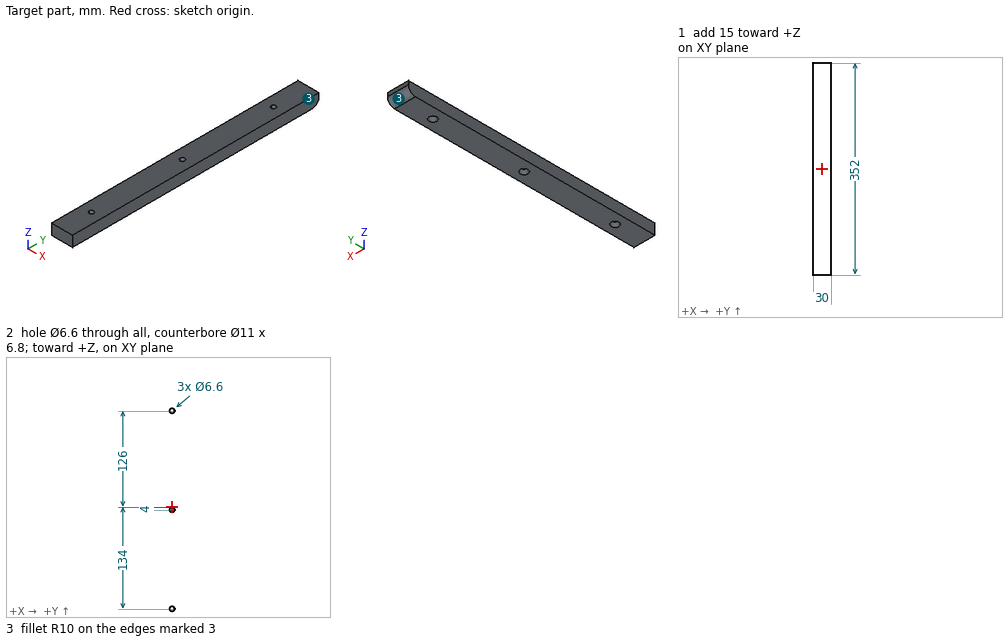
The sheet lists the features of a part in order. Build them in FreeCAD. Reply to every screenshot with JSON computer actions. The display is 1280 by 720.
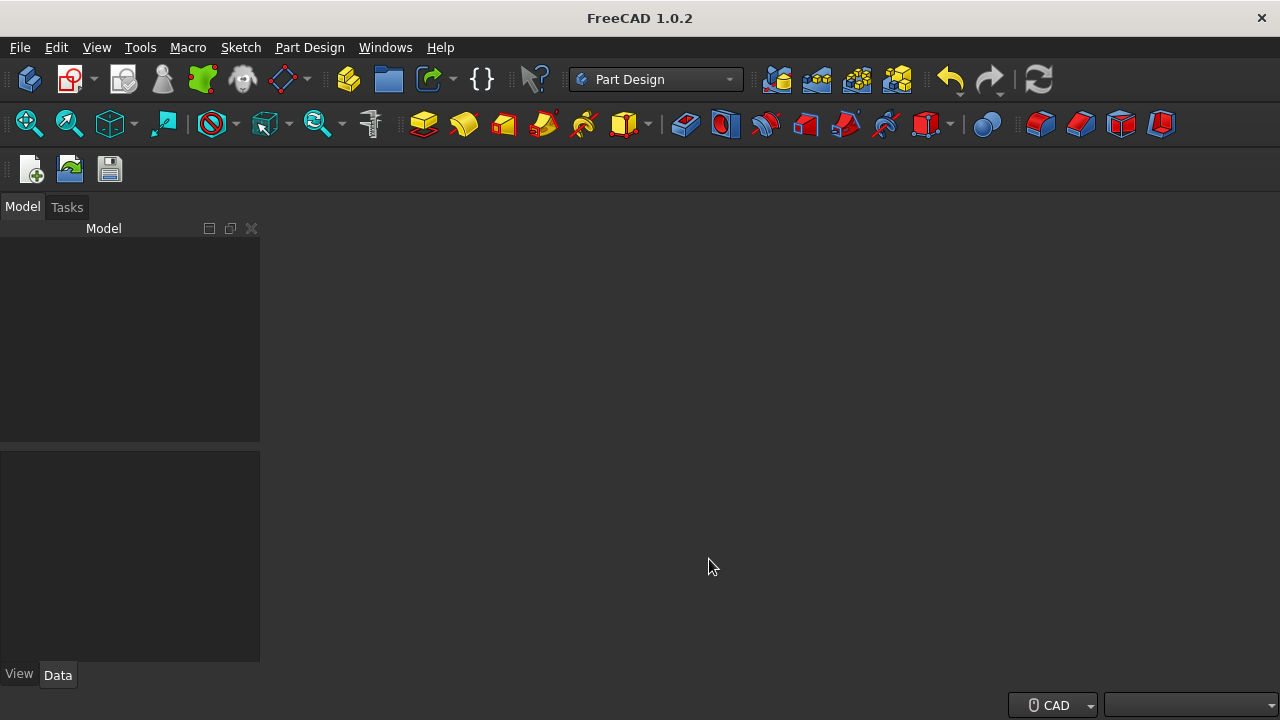
{"action": "left_click", "coordinate": [30, 170]}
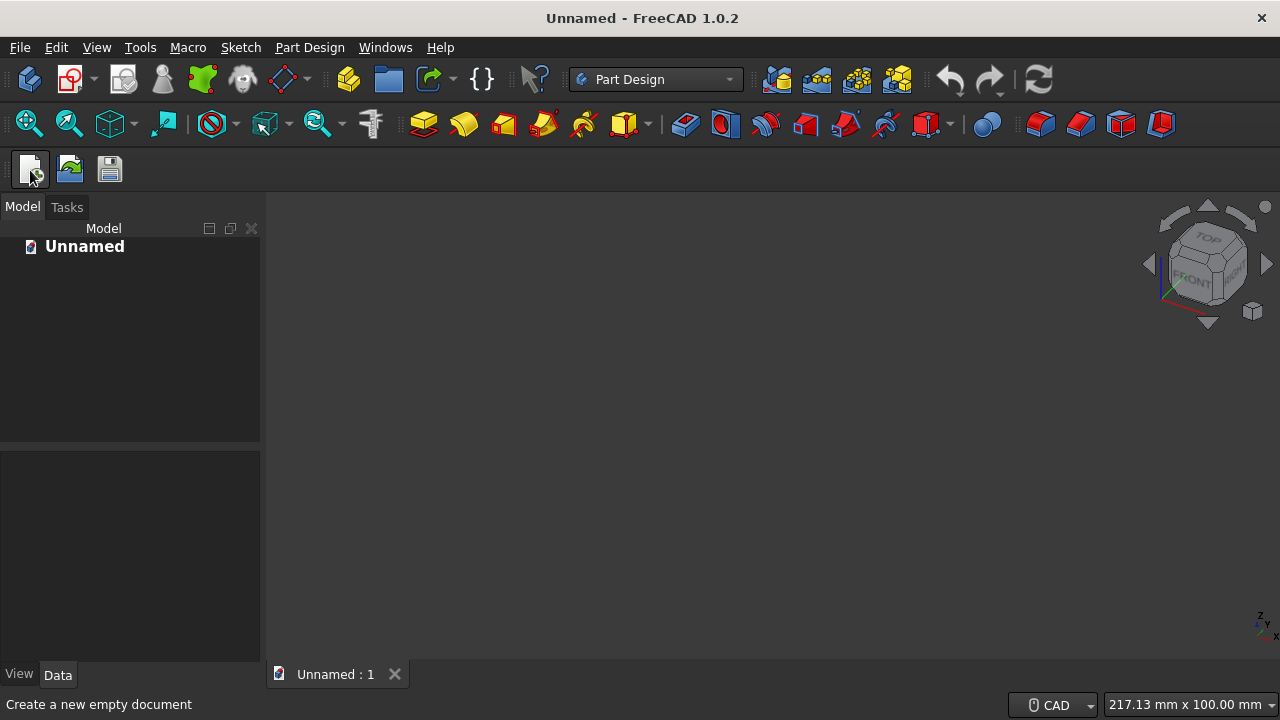
{"action": "left_click", "coordinate": [70, 80]}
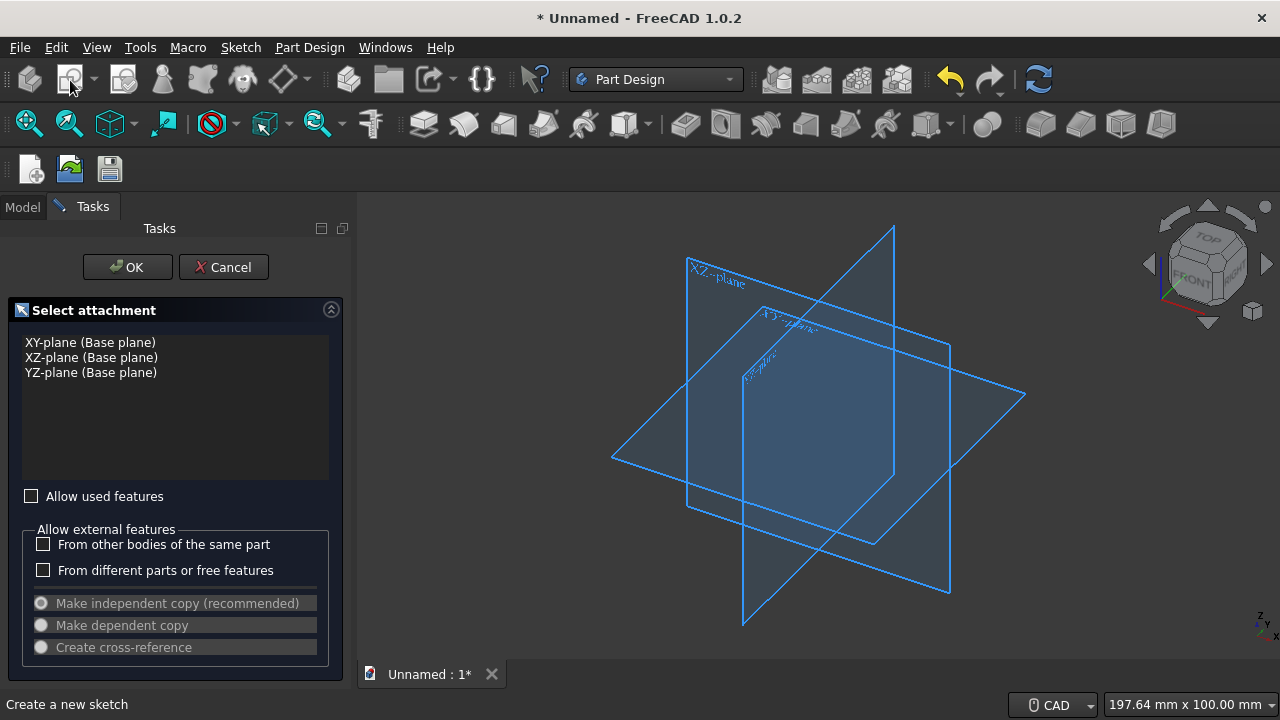
{"action": "left_click", "coordinate": [82, 342]}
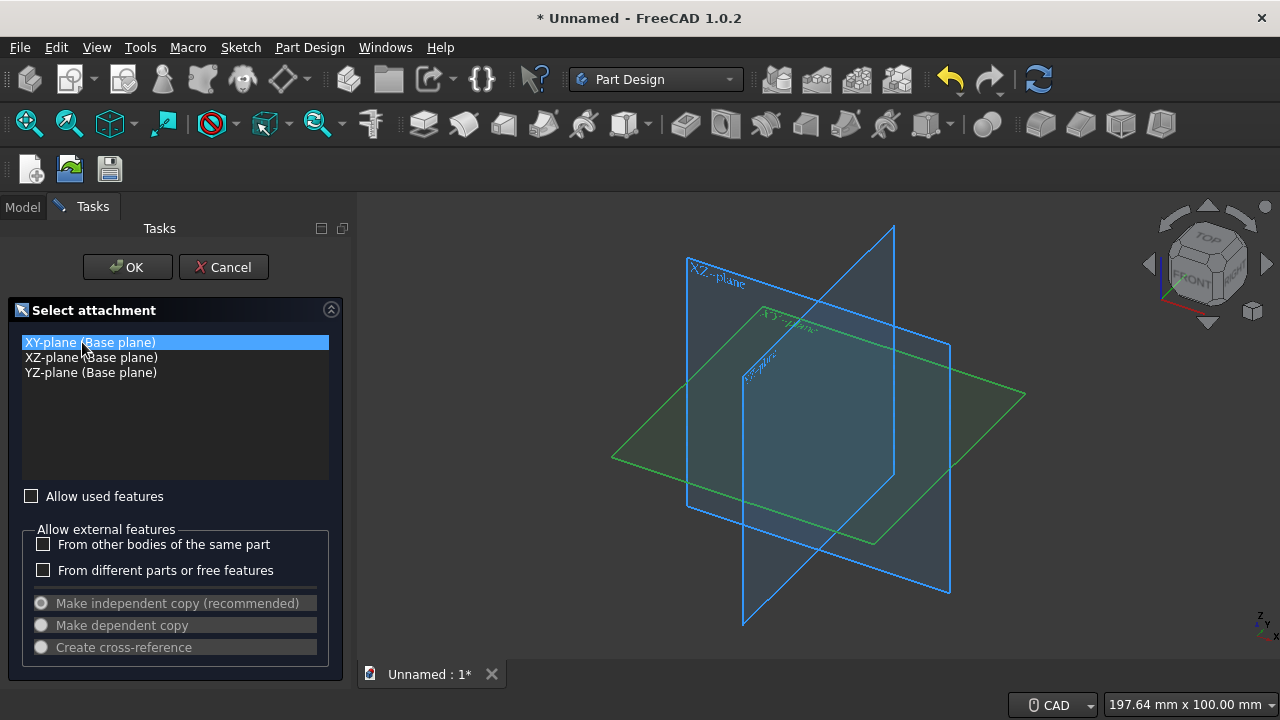
{"action": "left_click", "coordinate": [128, 267]}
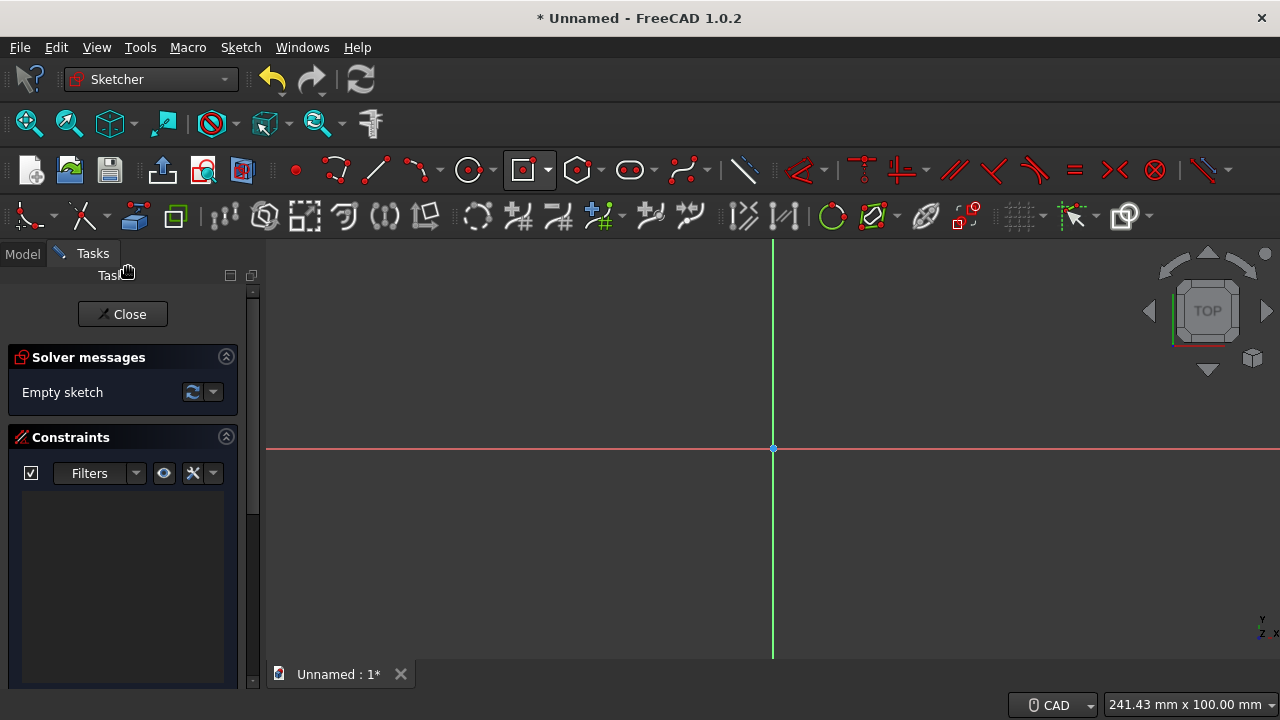
{"action": "scroll", "coordinate": [691, 449], "scroll_direction": "down", "scroll_amount": 9}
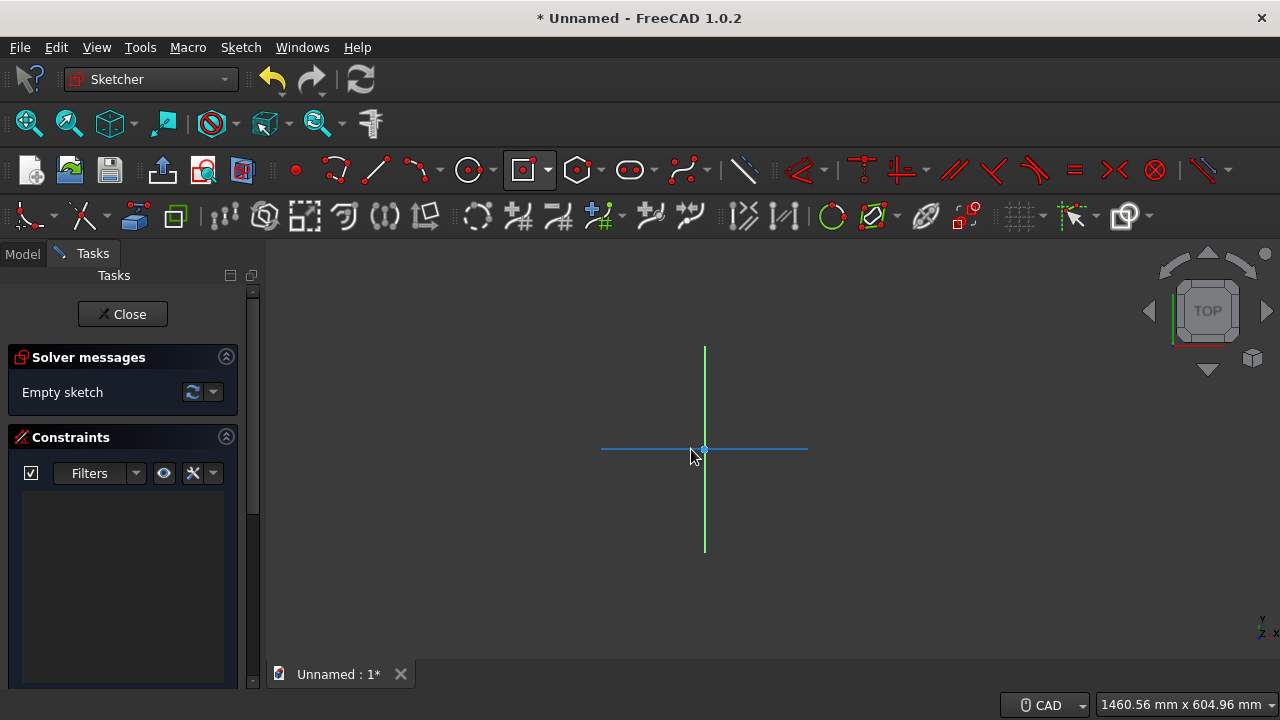
{"action": "left_click", "coordinate": [524, 170]}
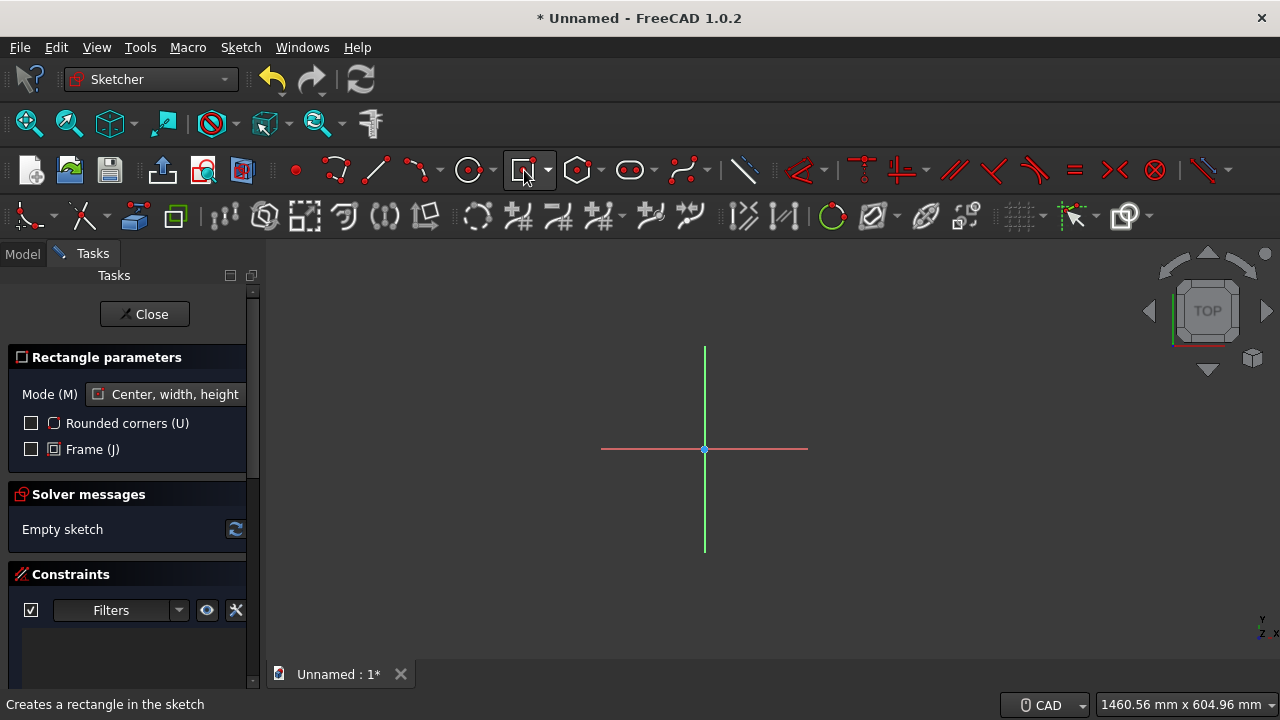
{"action": "scroll", "coordinate": [705, 449], "scroll_direction": "up", "scroll_amount": 3}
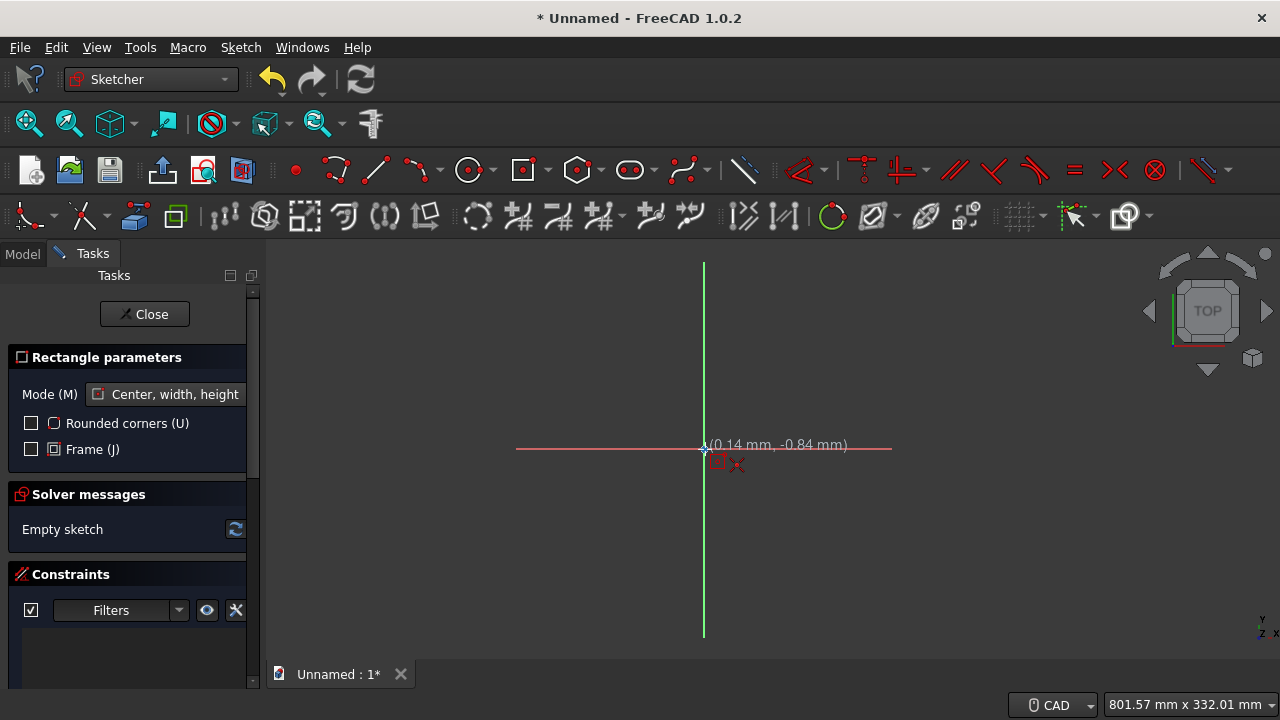
{"action": "left_click", "coordinate": [704, 449]}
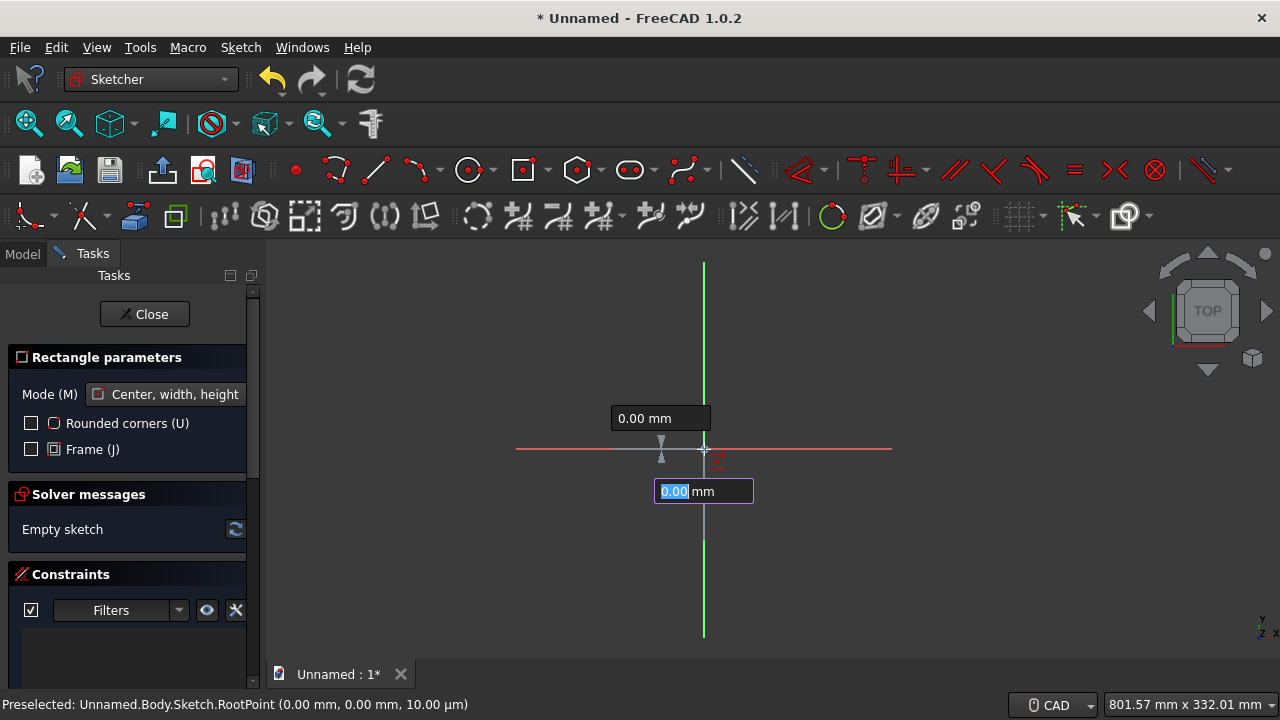
{"action": "scroll", "coordinate": [705, 449], "scroll_direction": "down", "scroll_amount": 3}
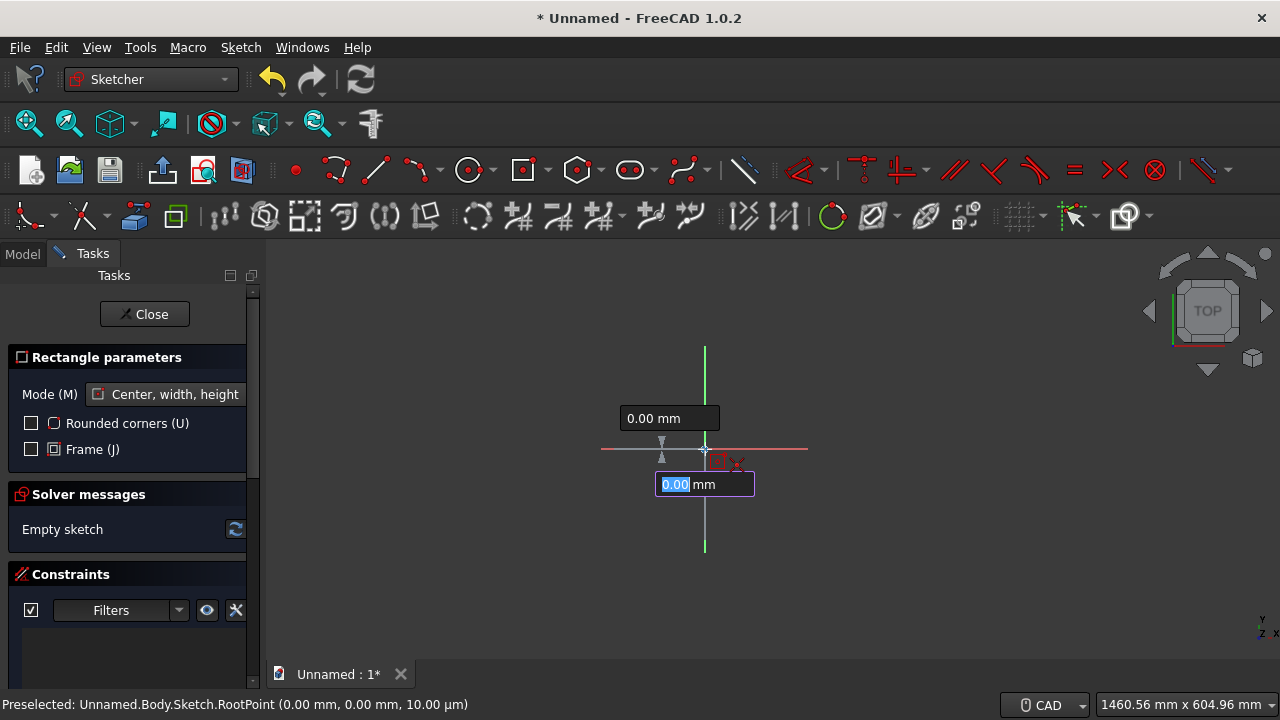
{"action": "scroll", "coordinate": [715, 327], "scroll_direction": "up", "scroll_amount": 3}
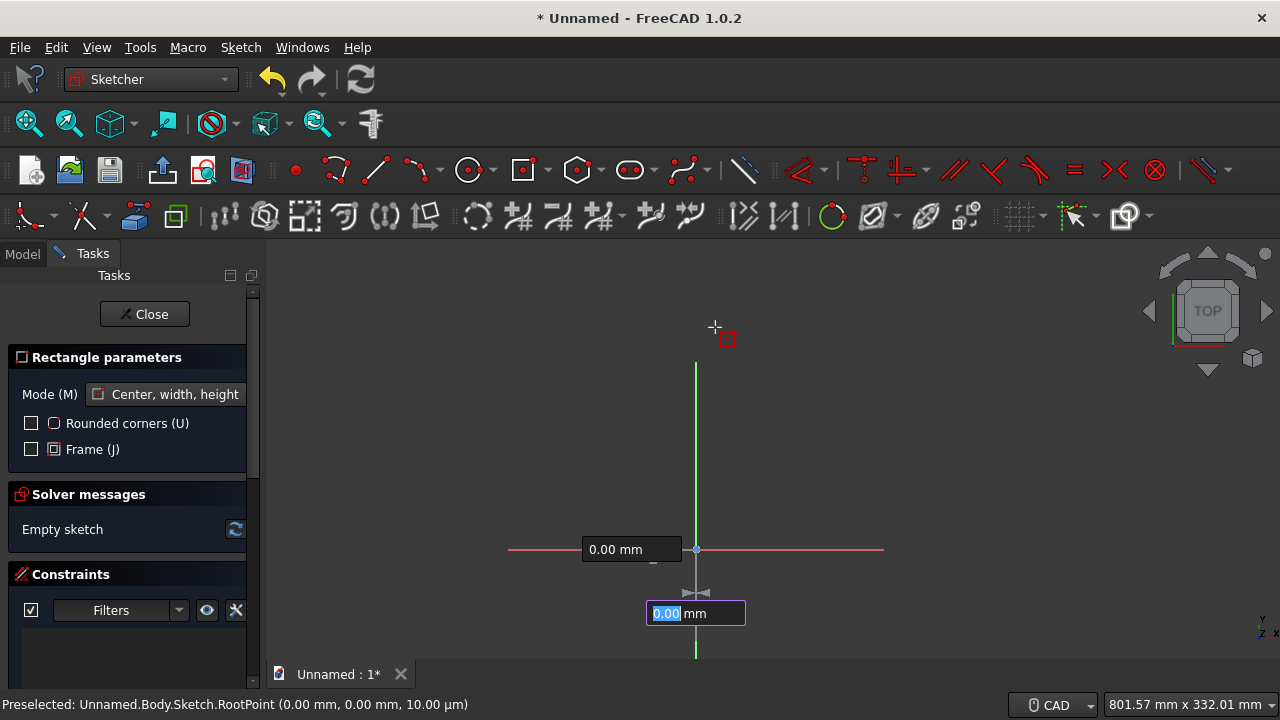
{"action": "left_click", "coordinate": [715, 327]}
{"action": "key", "text": "Escape"}